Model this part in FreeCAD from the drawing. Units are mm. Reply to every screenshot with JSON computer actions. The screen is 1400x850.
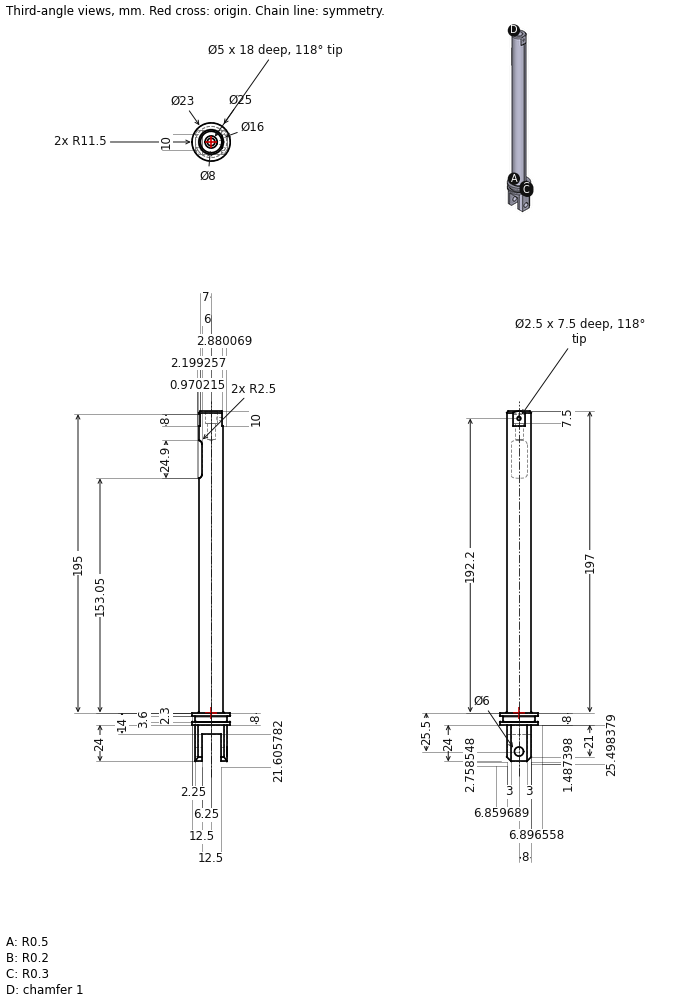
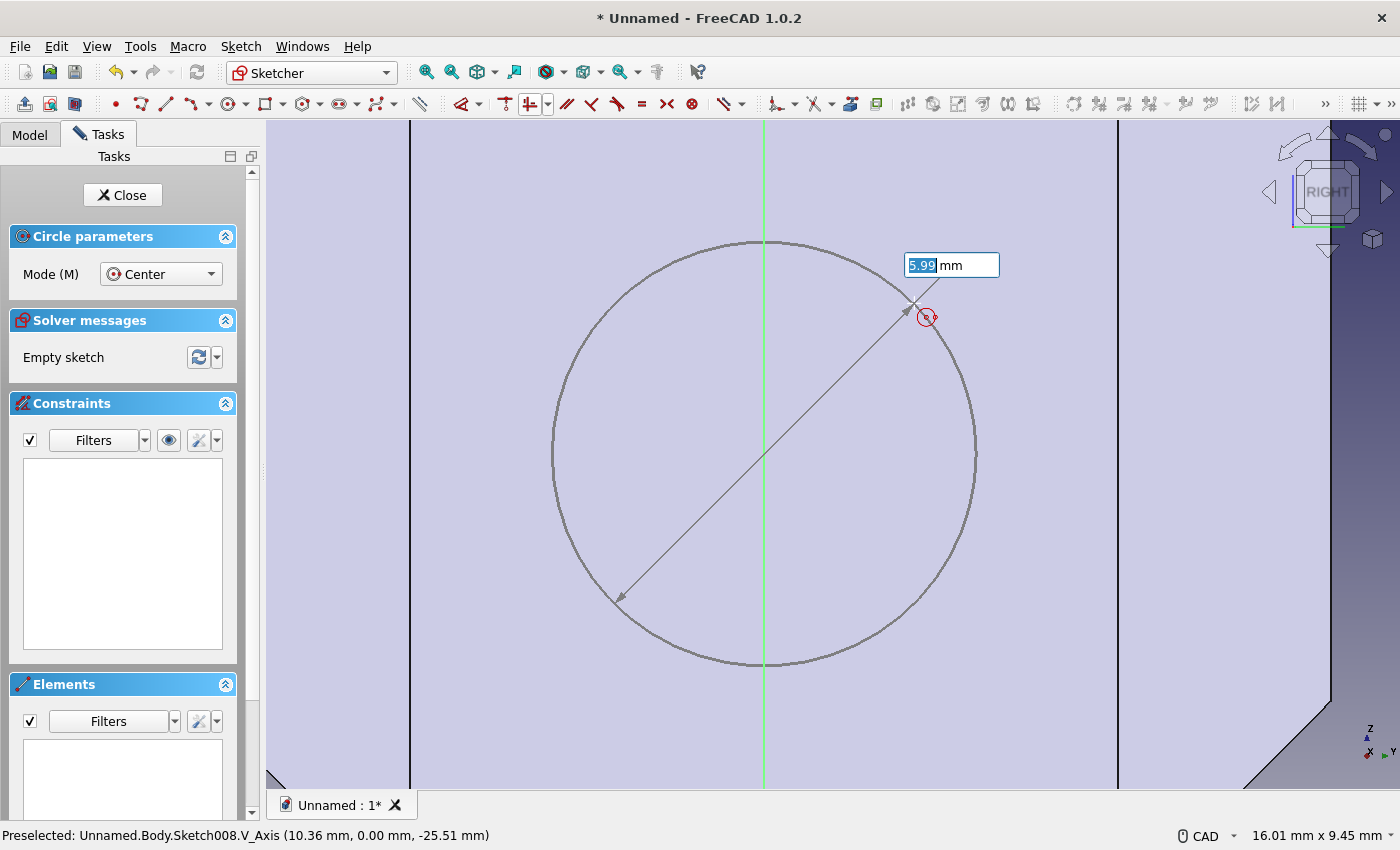
{"action": "type", "text": "6"}
{"action": "key", "text": "Return"}
{"action": "key", "text": "Escape"}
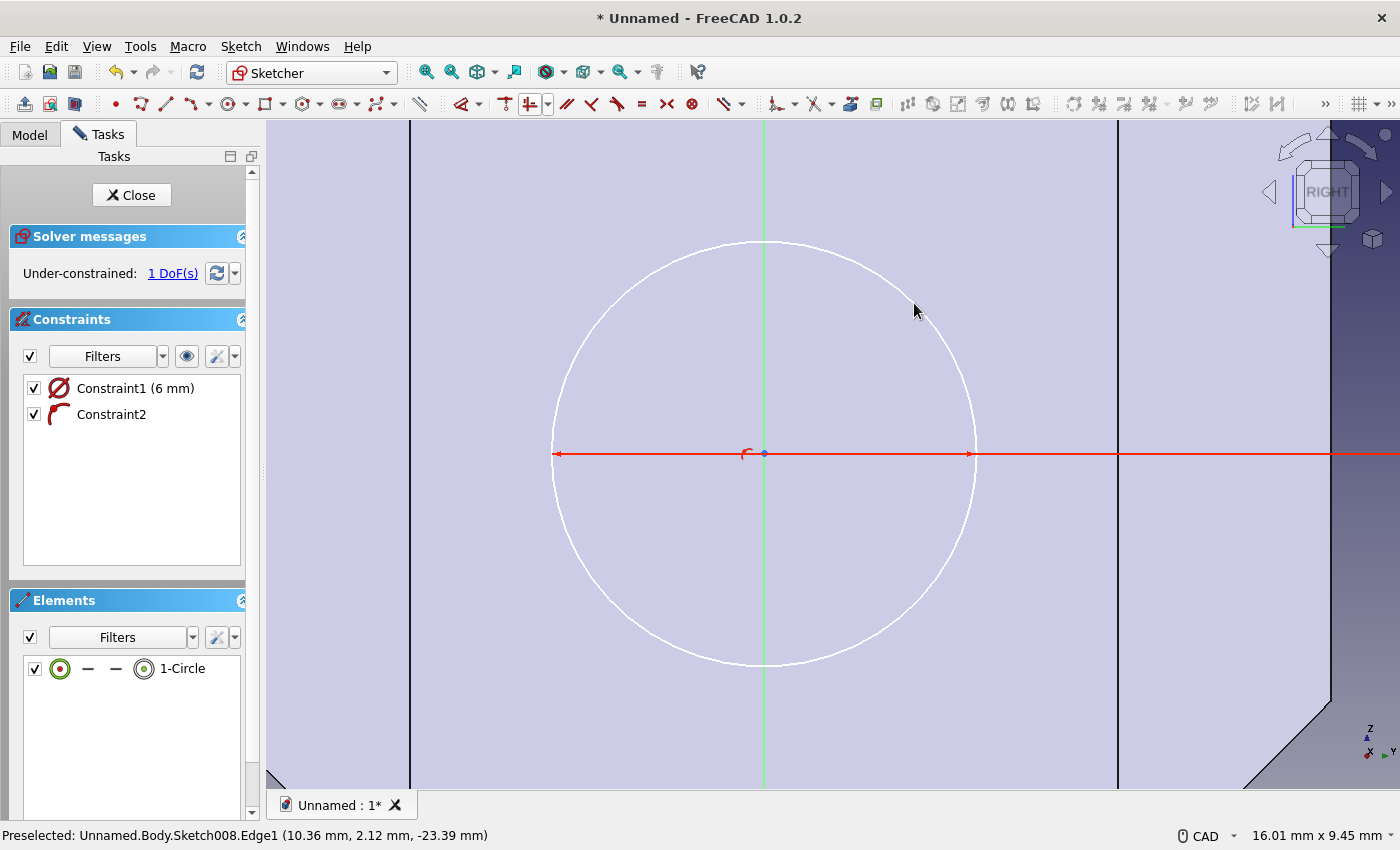
{"action": "left_click", "coordinate": [460, 104]}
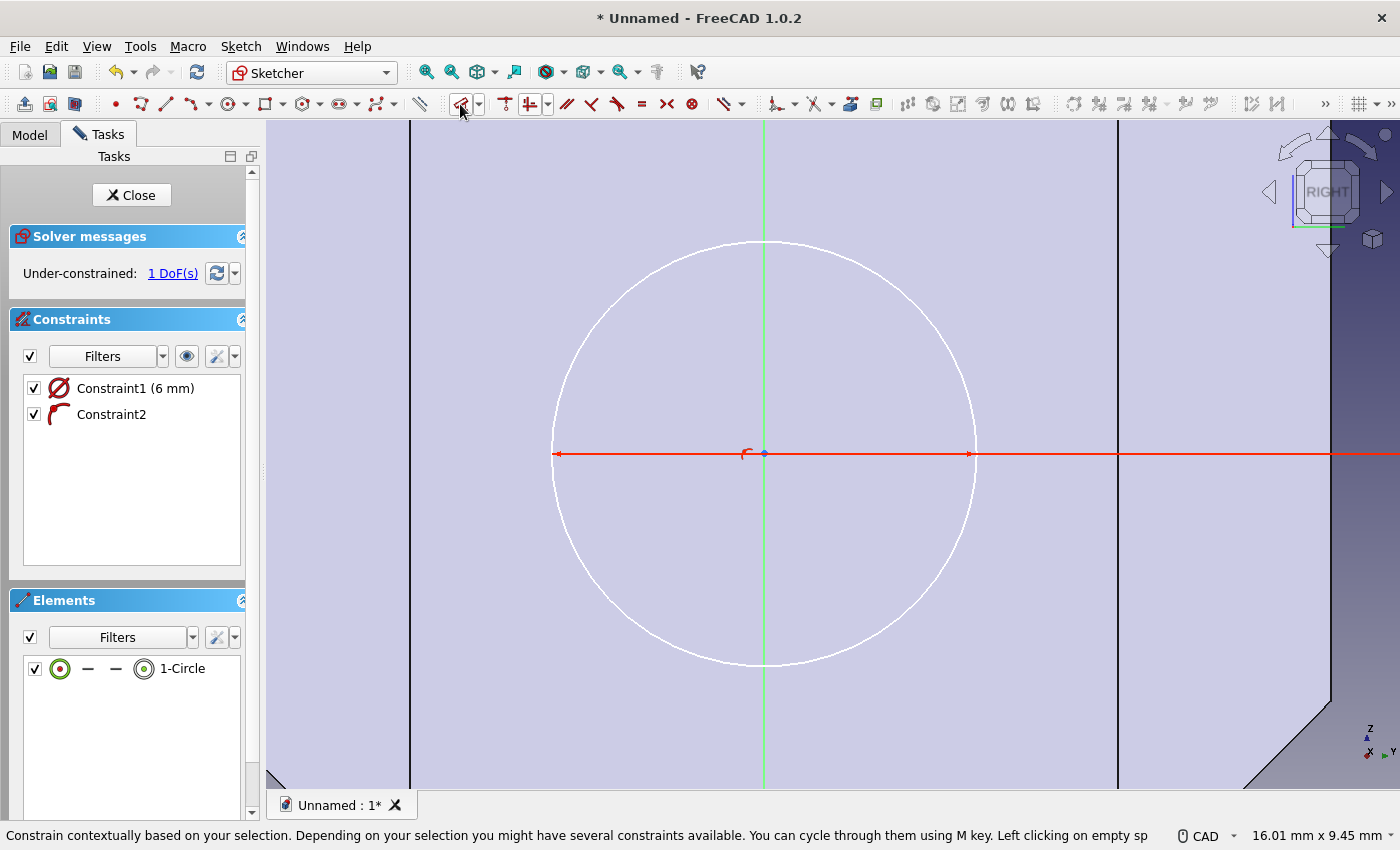
{"action": "left_click", "coordinate": [764, 454]}
{"action": "left_click", "coordinate": [798, 301]}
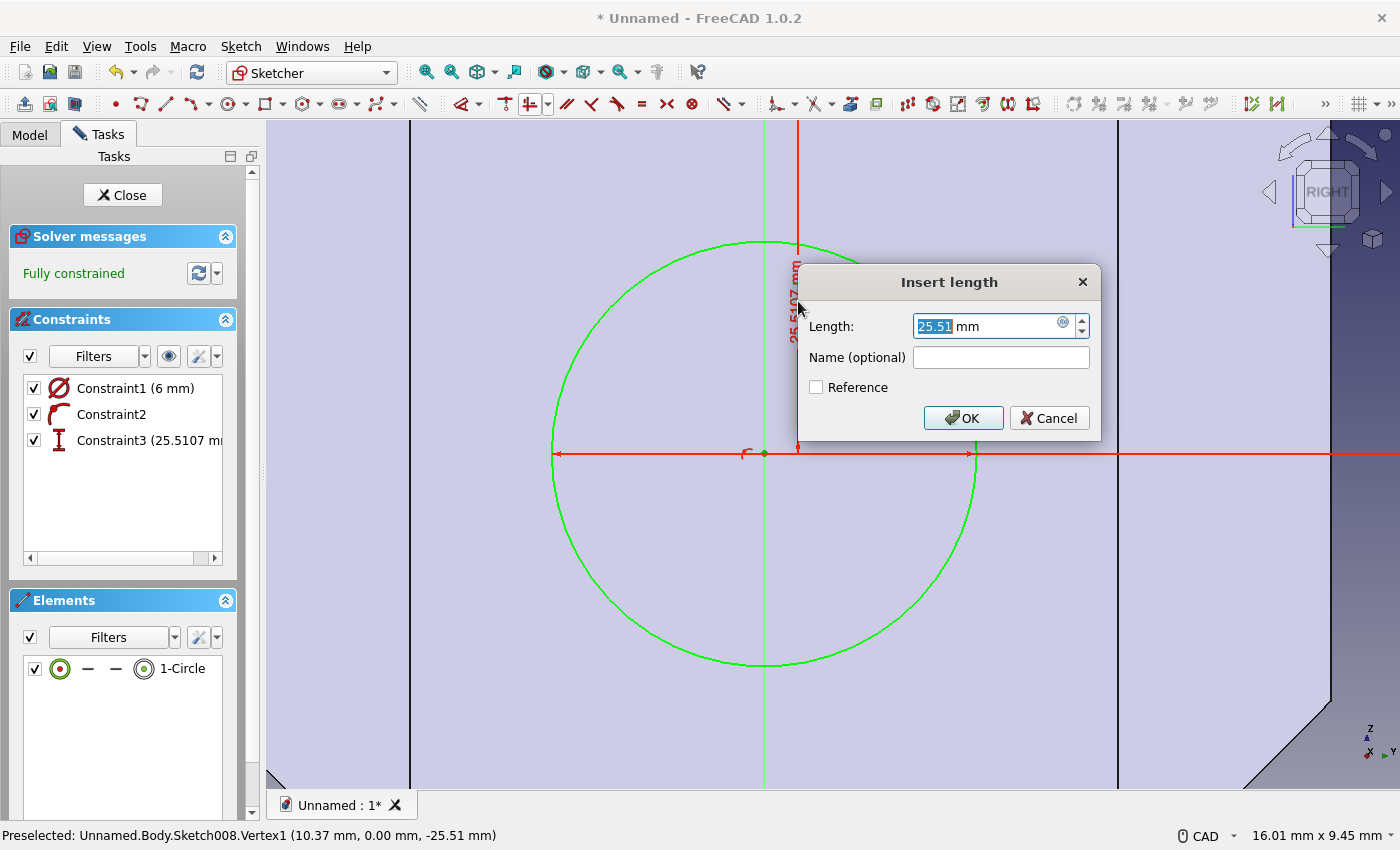
{"action": "type", "text": "25.5"}
{"action": "key", "text": "Return"}
{"action": "key", "text": "Escape"}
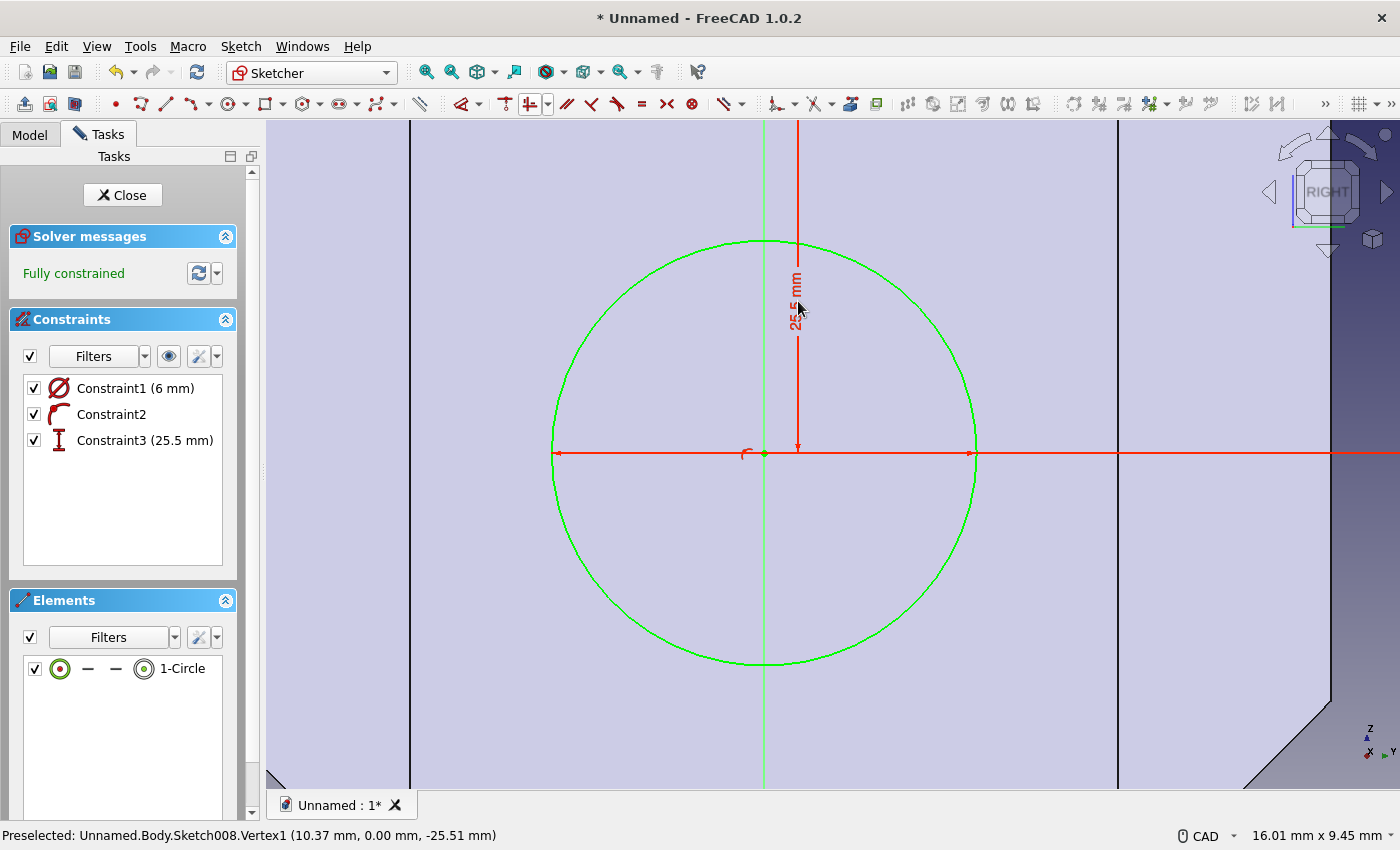
{"action": "left_click", "coordinate": [123, 195]}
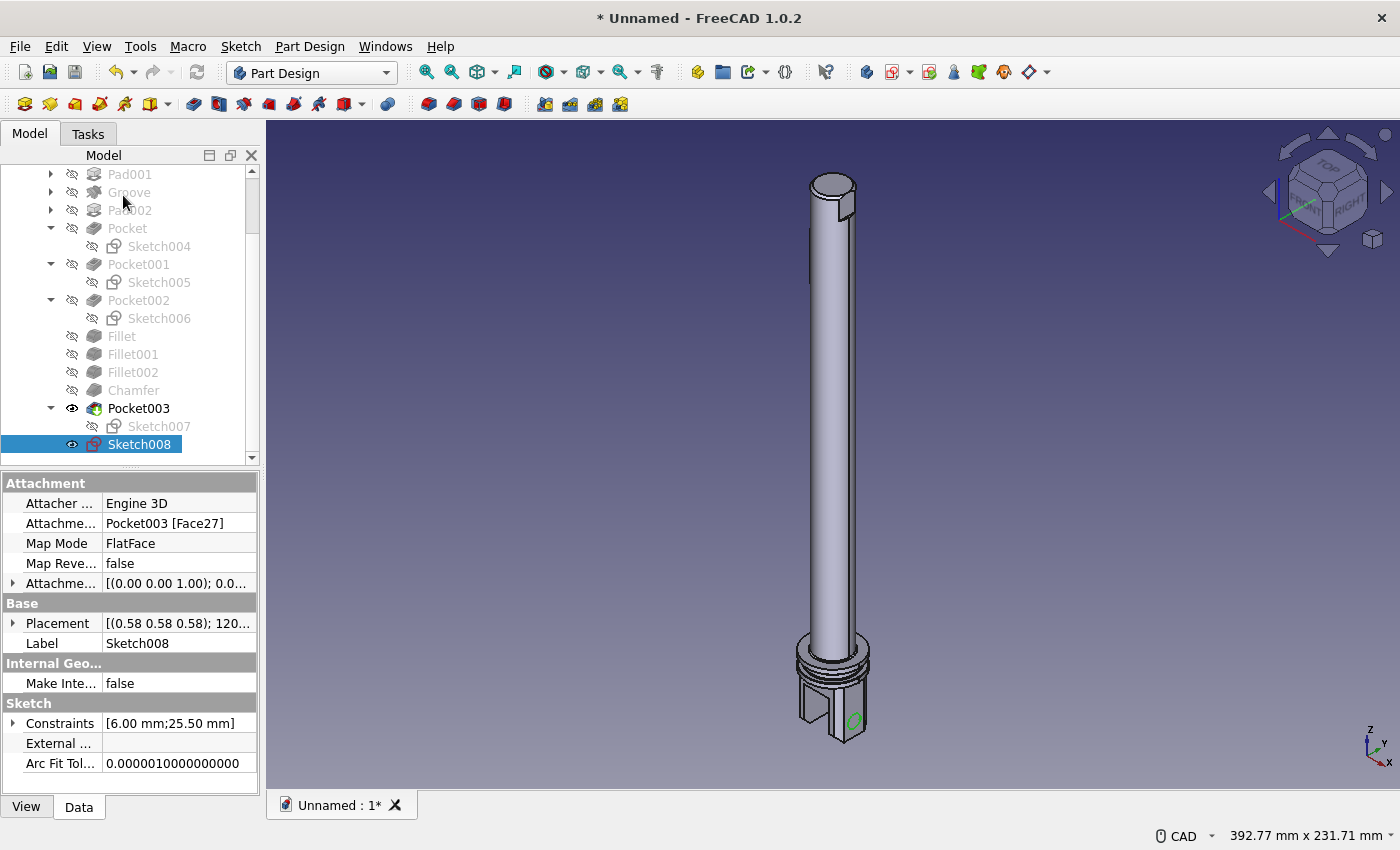
{"action": "left_click", "coordinate": [194, 104]}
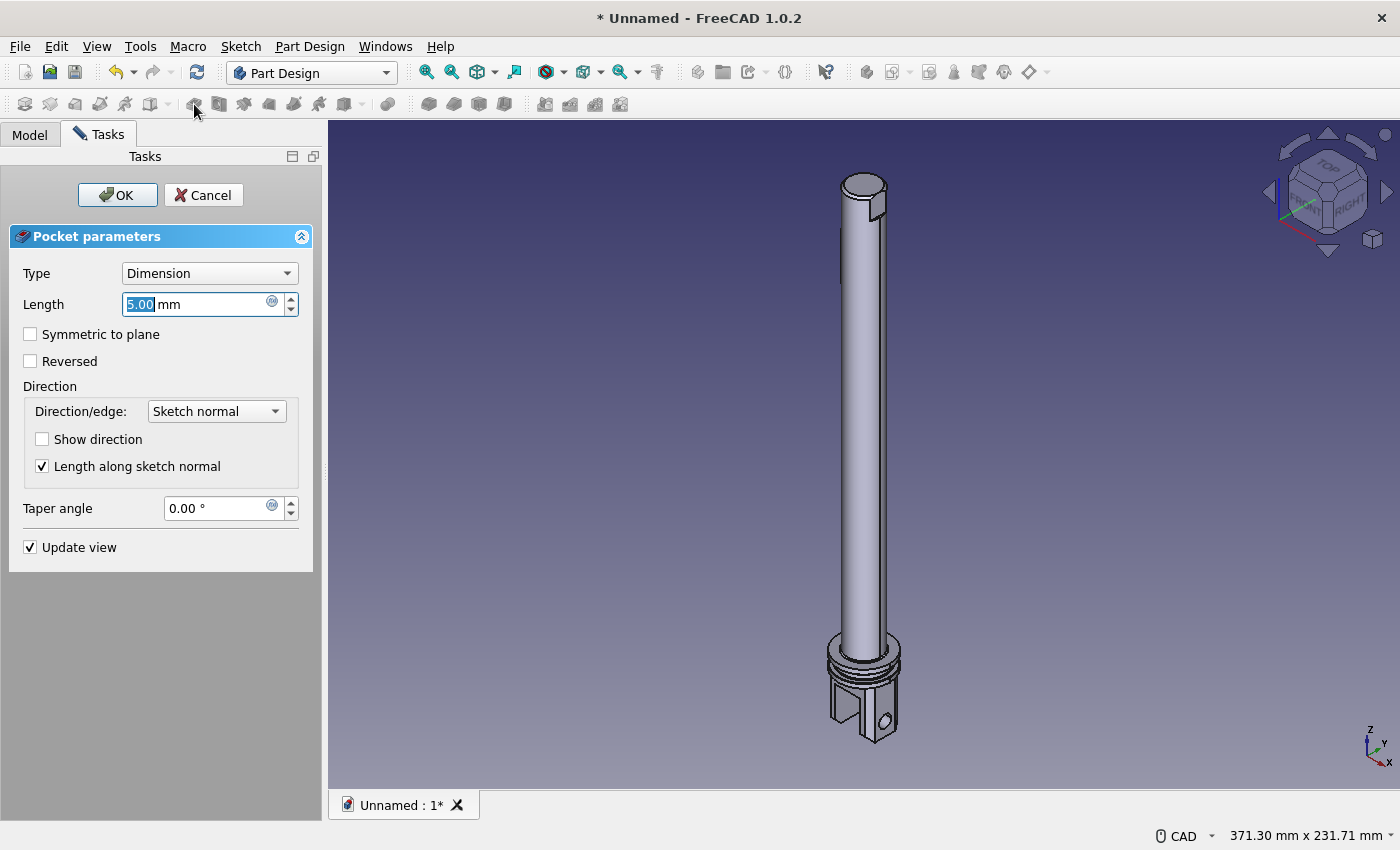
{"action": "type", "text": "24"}
{"action": "key", "text": "Tab"}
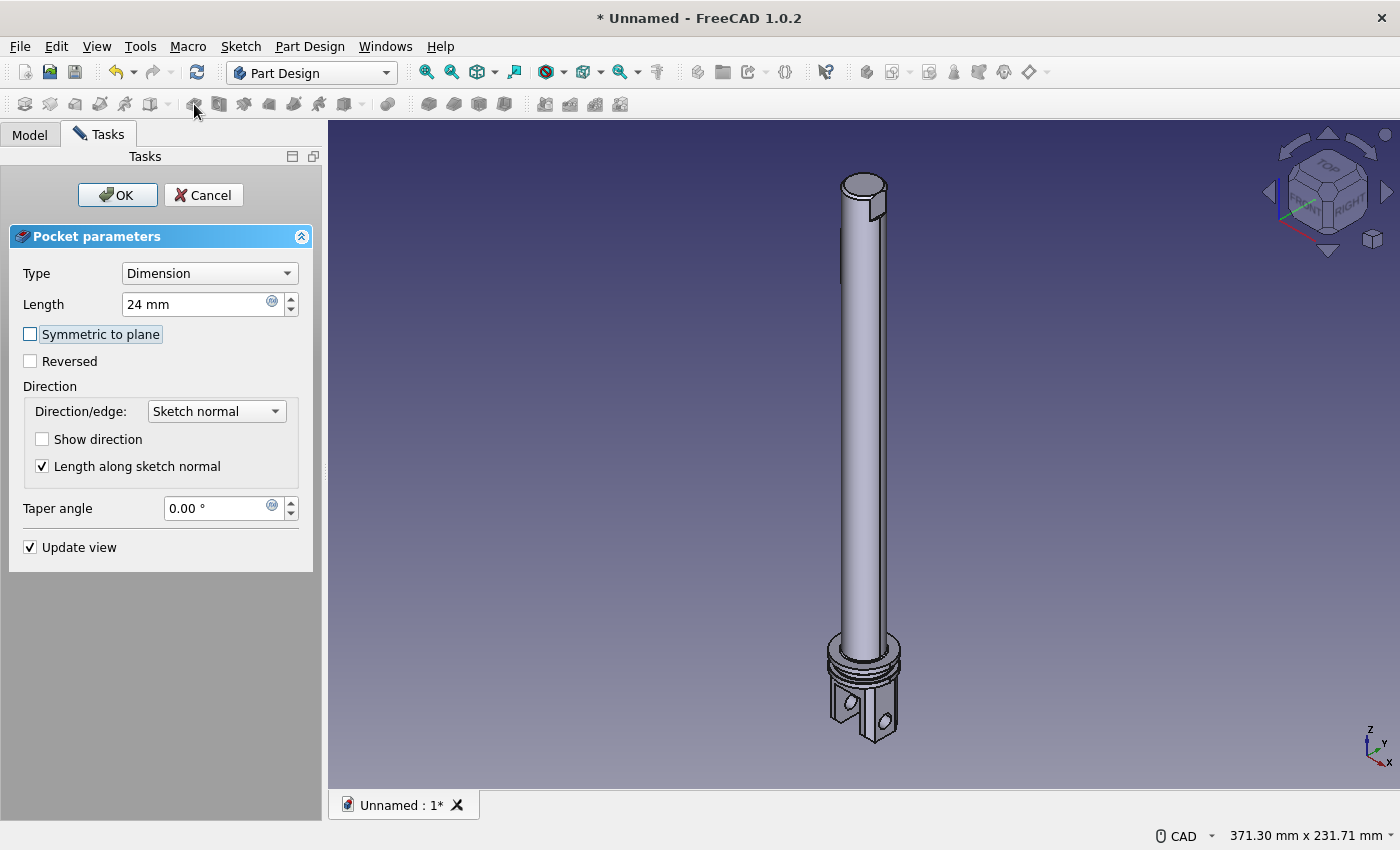
{"action": "left_click", "coordinate": [118, 195]}